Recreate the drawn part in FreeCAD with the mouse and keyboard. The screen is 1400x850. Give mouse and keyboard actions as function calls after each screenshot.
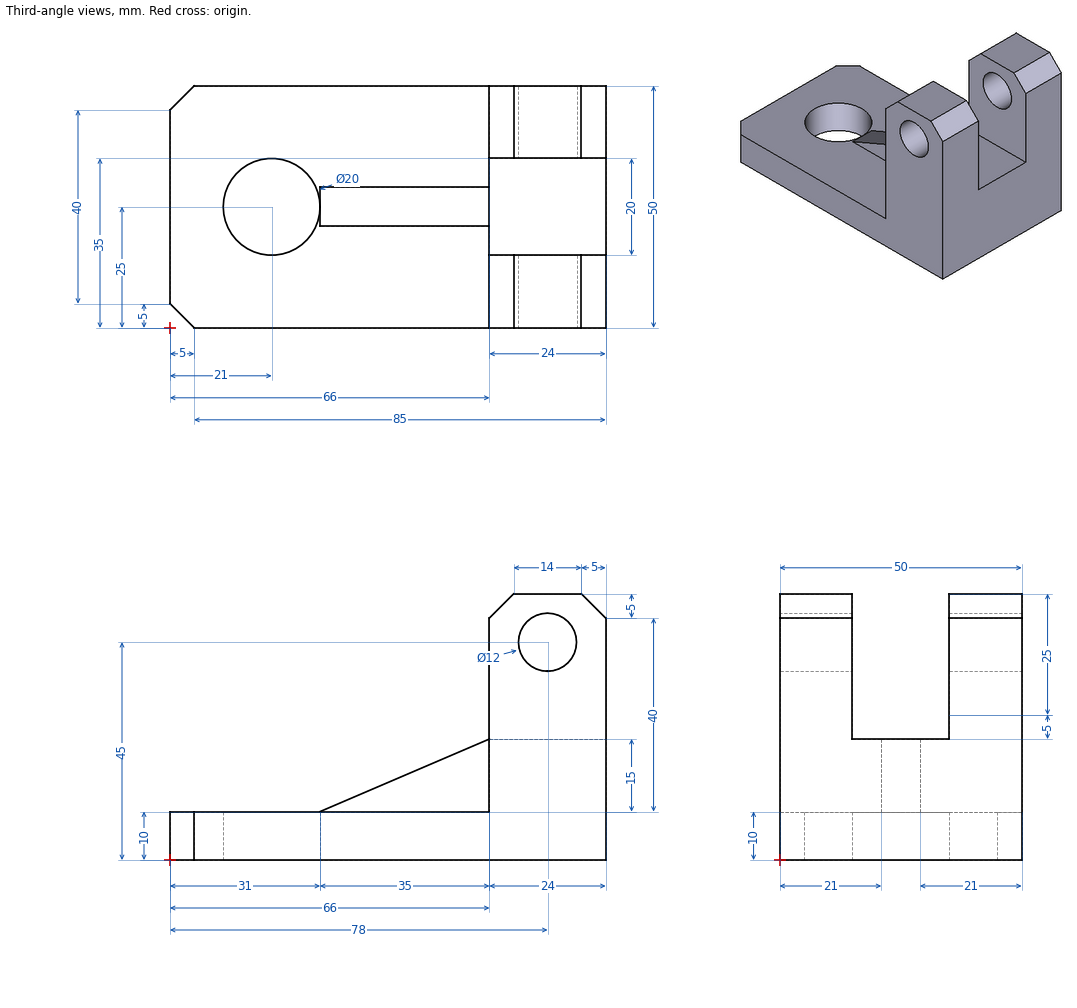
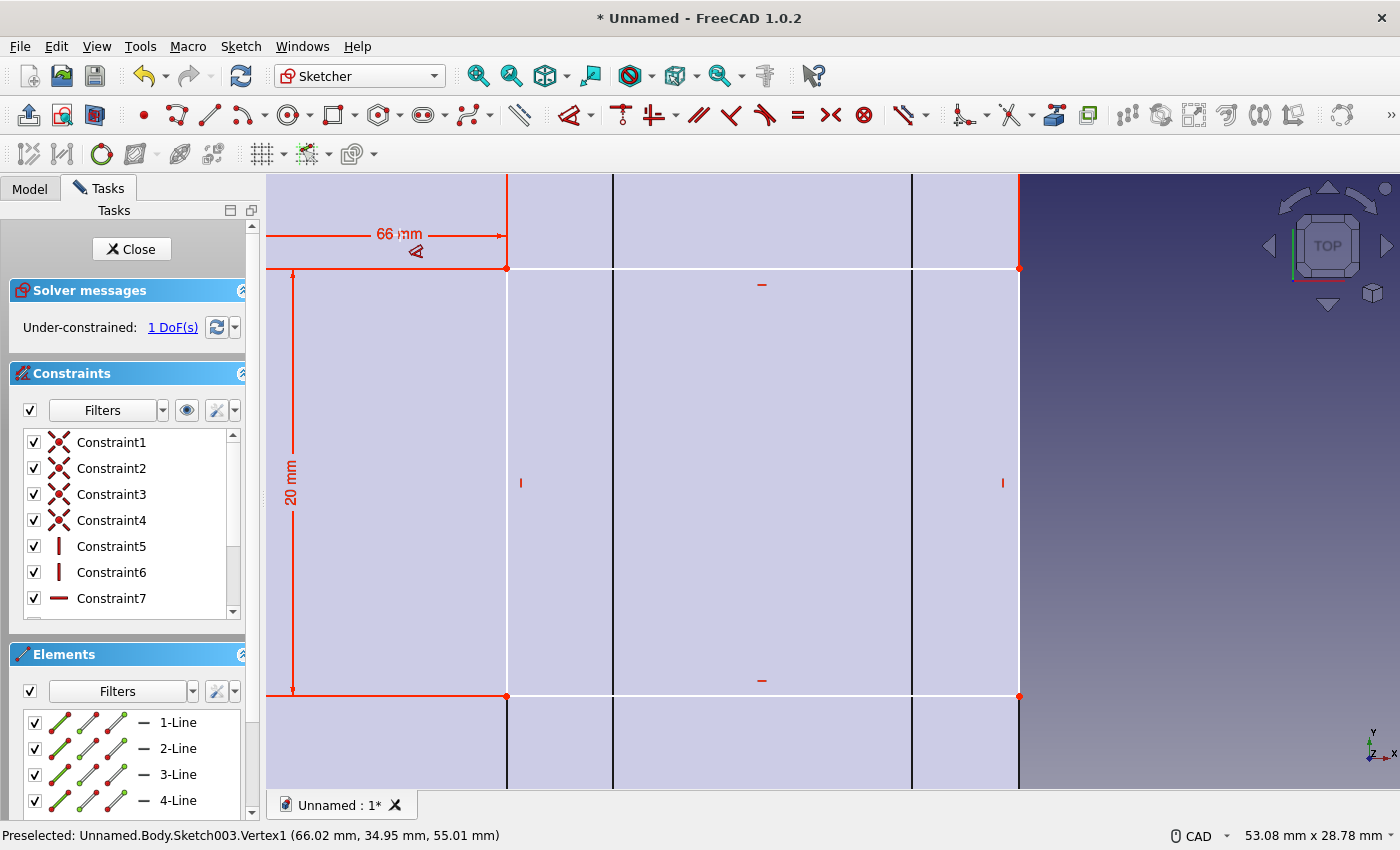
click(507, 269)
click(541, 515)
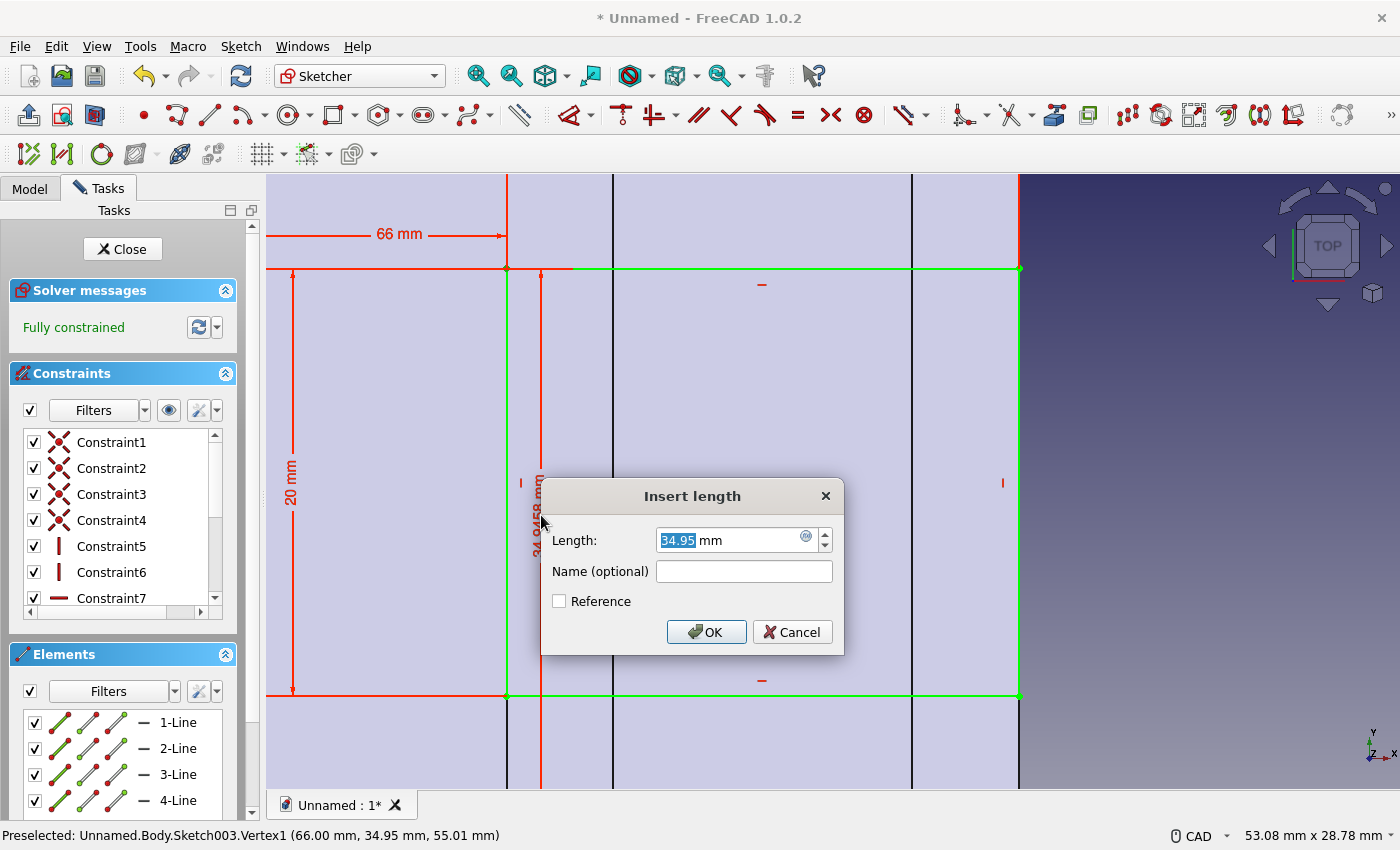
text(35)
key(Return)
key(Escape)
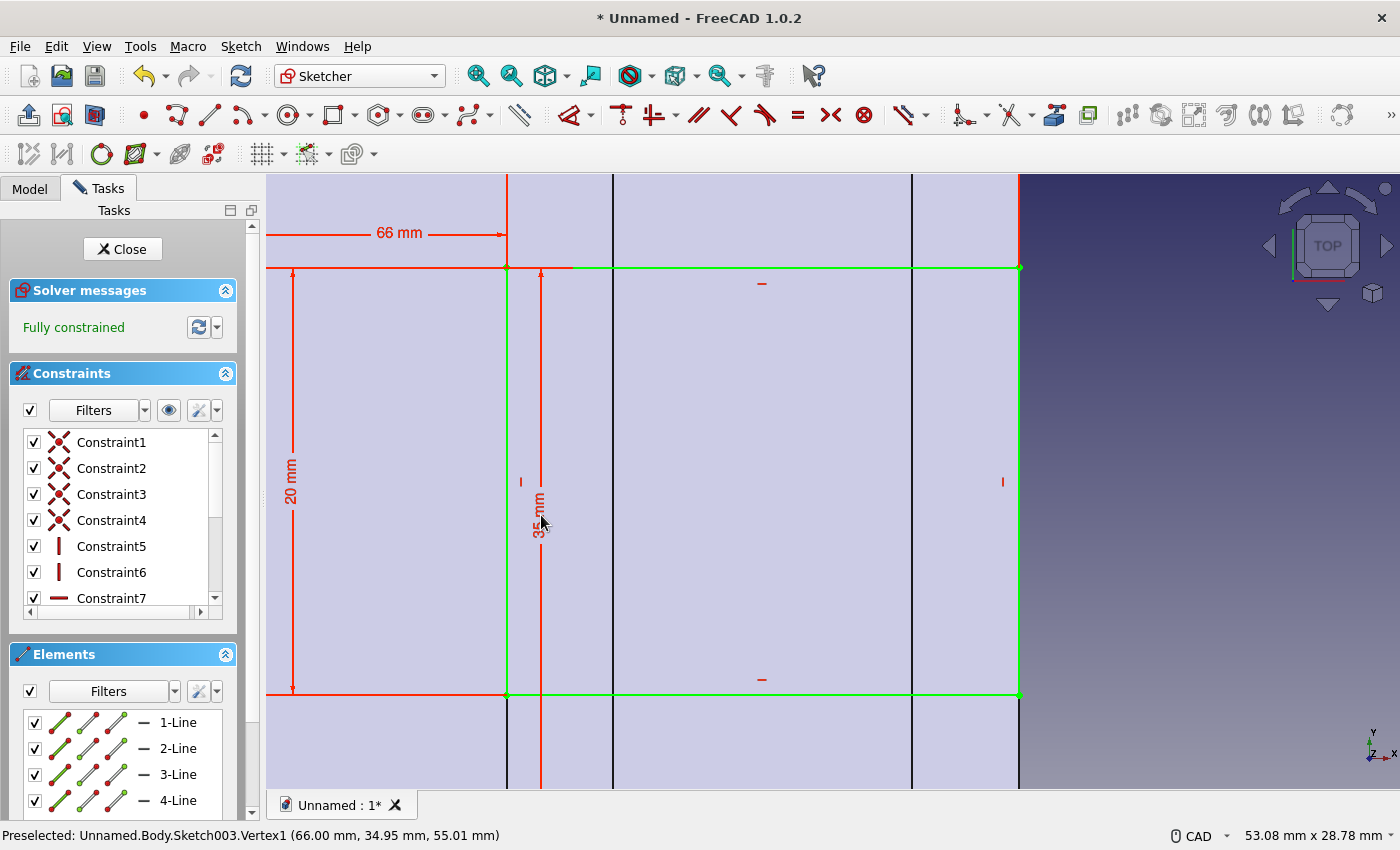
click(123, 249)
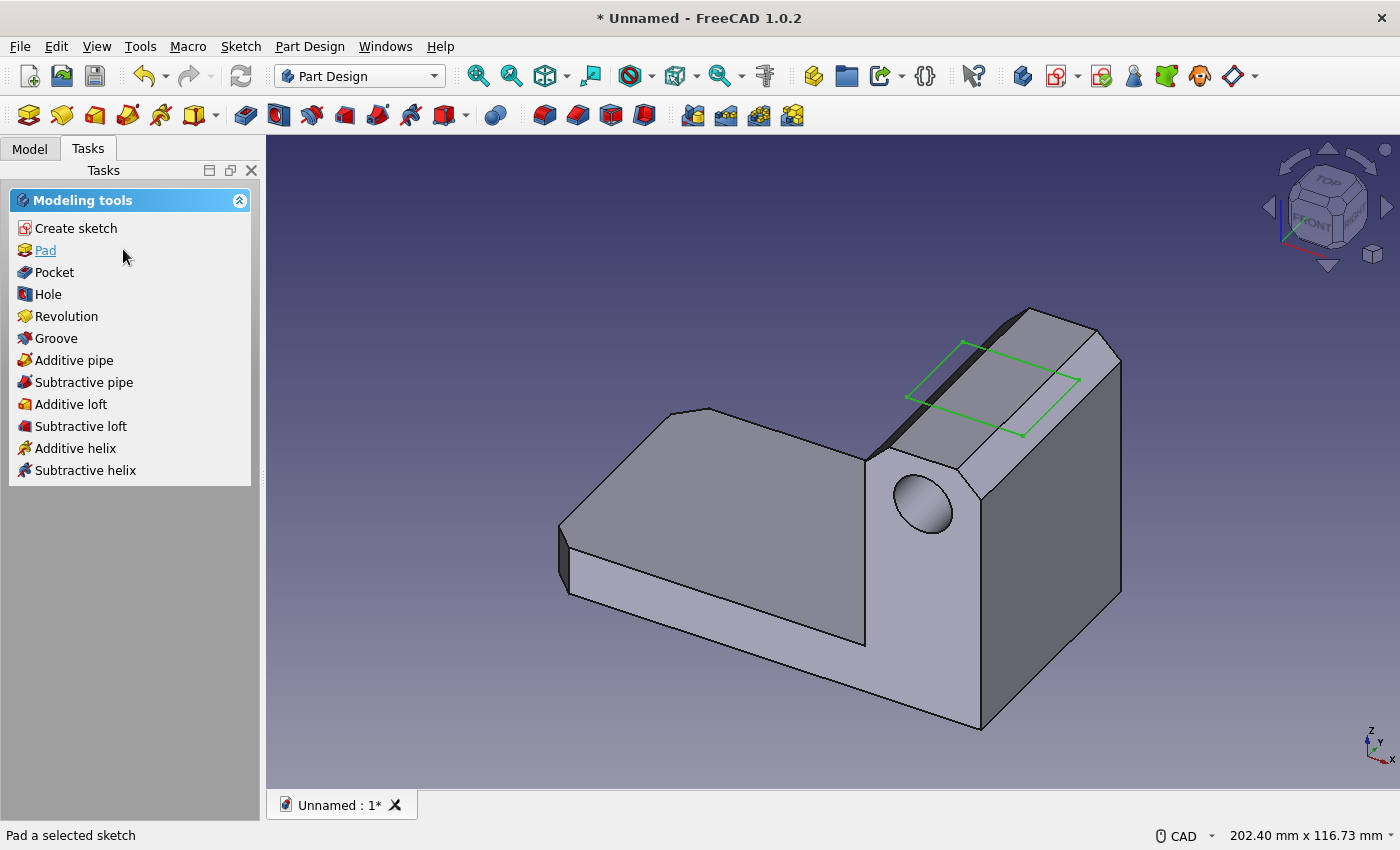
click(246, 116)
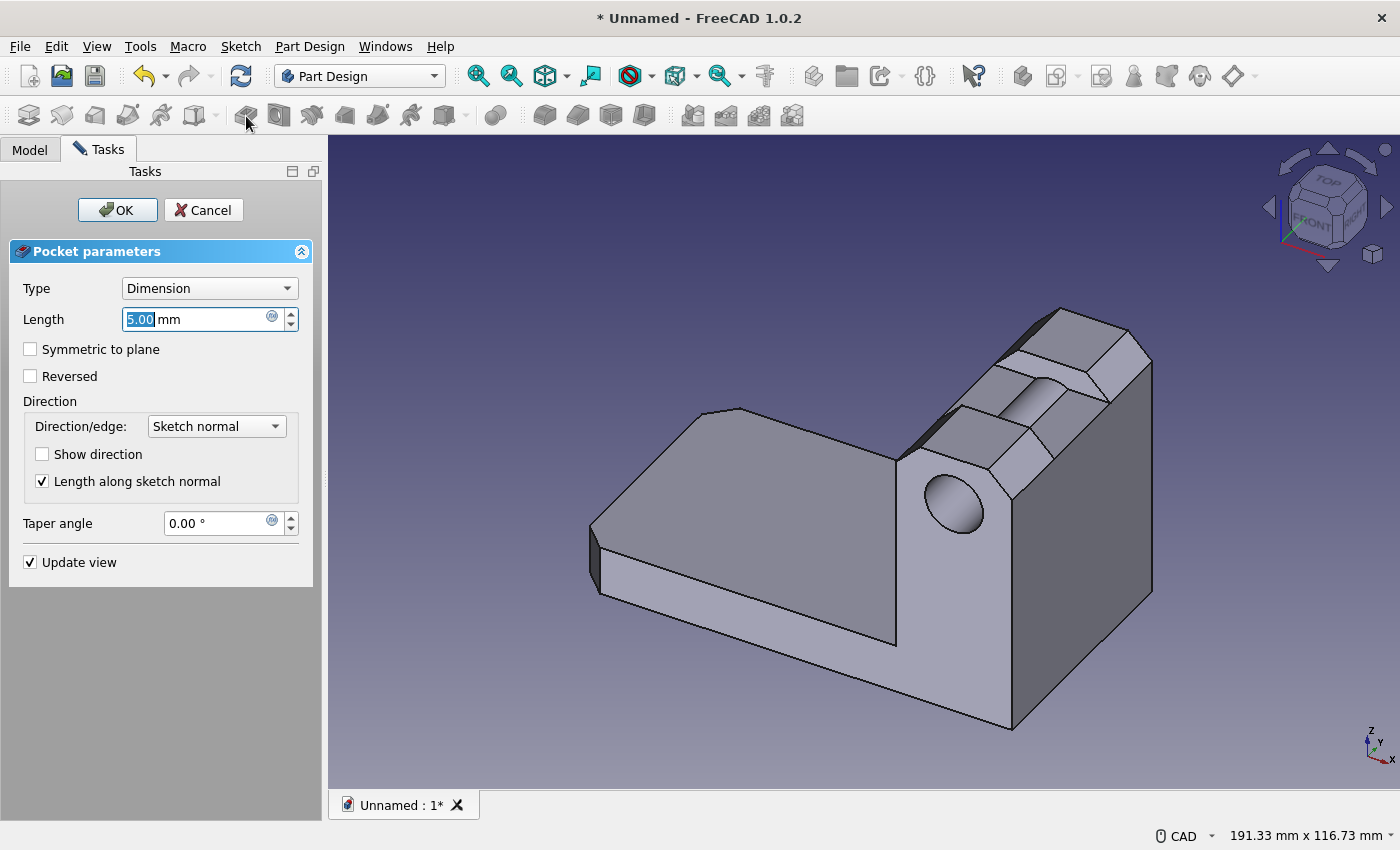
text(25)
key(Tab)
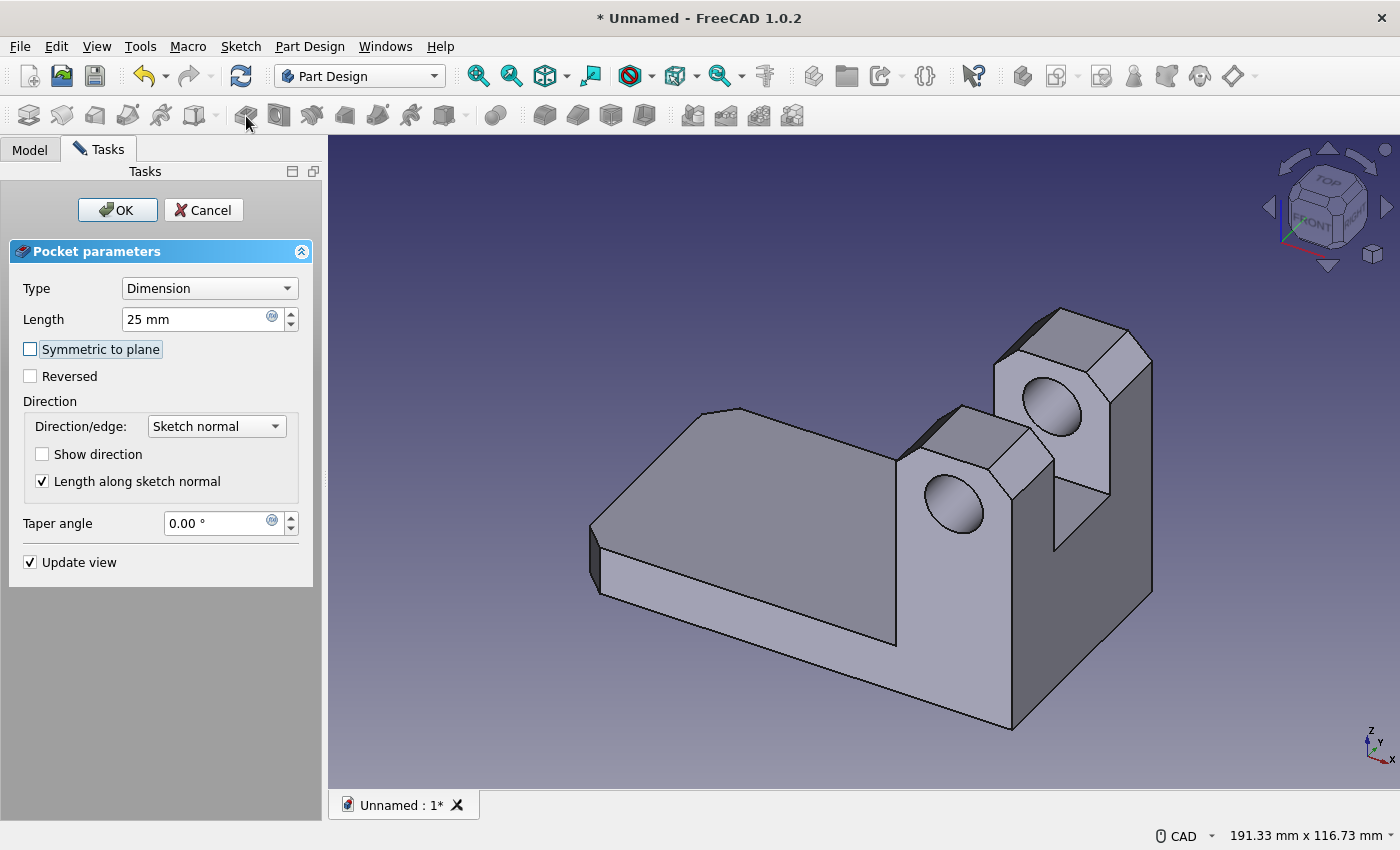
click(118, 210)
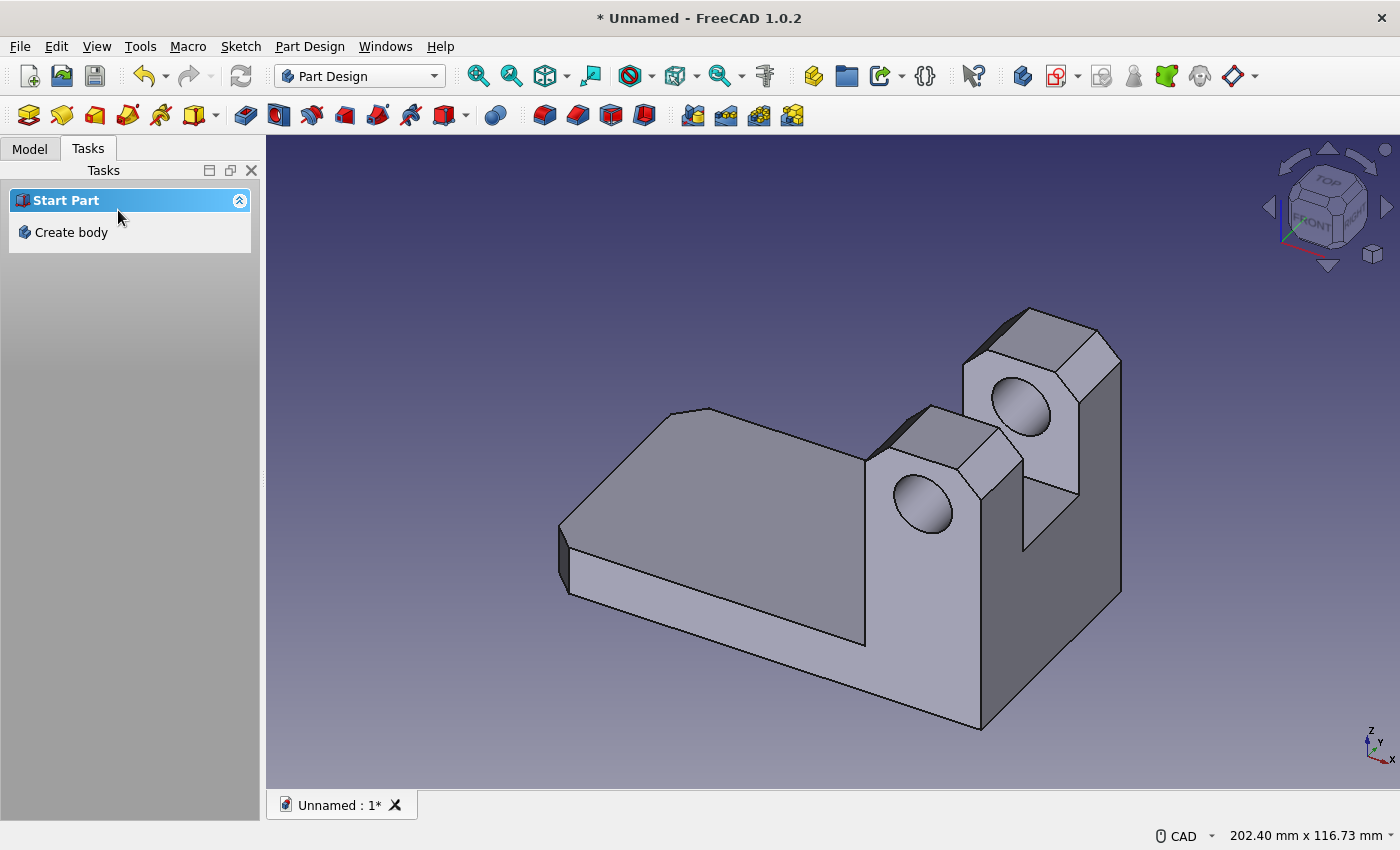
click(775, 522)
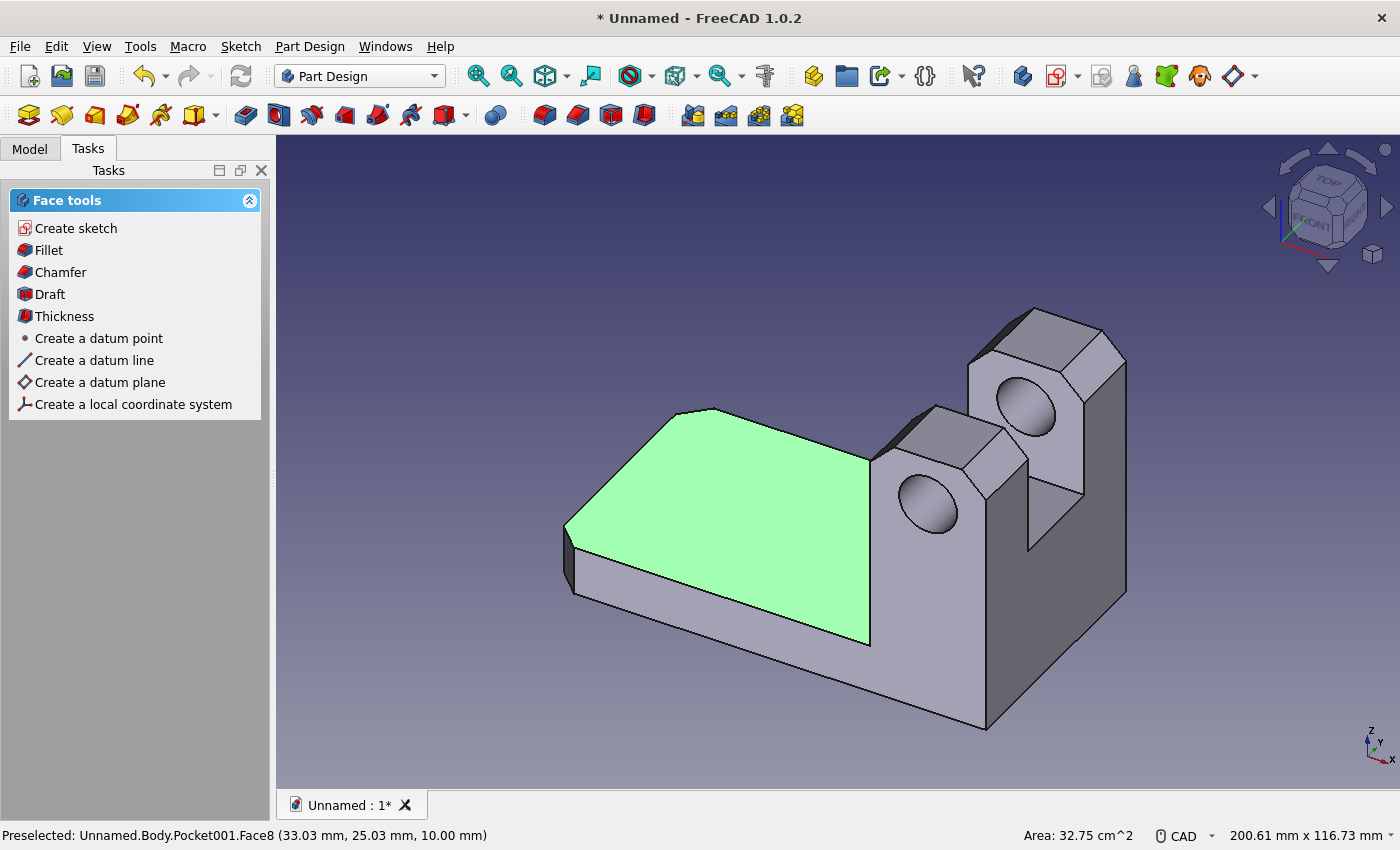
click(1056, 76)